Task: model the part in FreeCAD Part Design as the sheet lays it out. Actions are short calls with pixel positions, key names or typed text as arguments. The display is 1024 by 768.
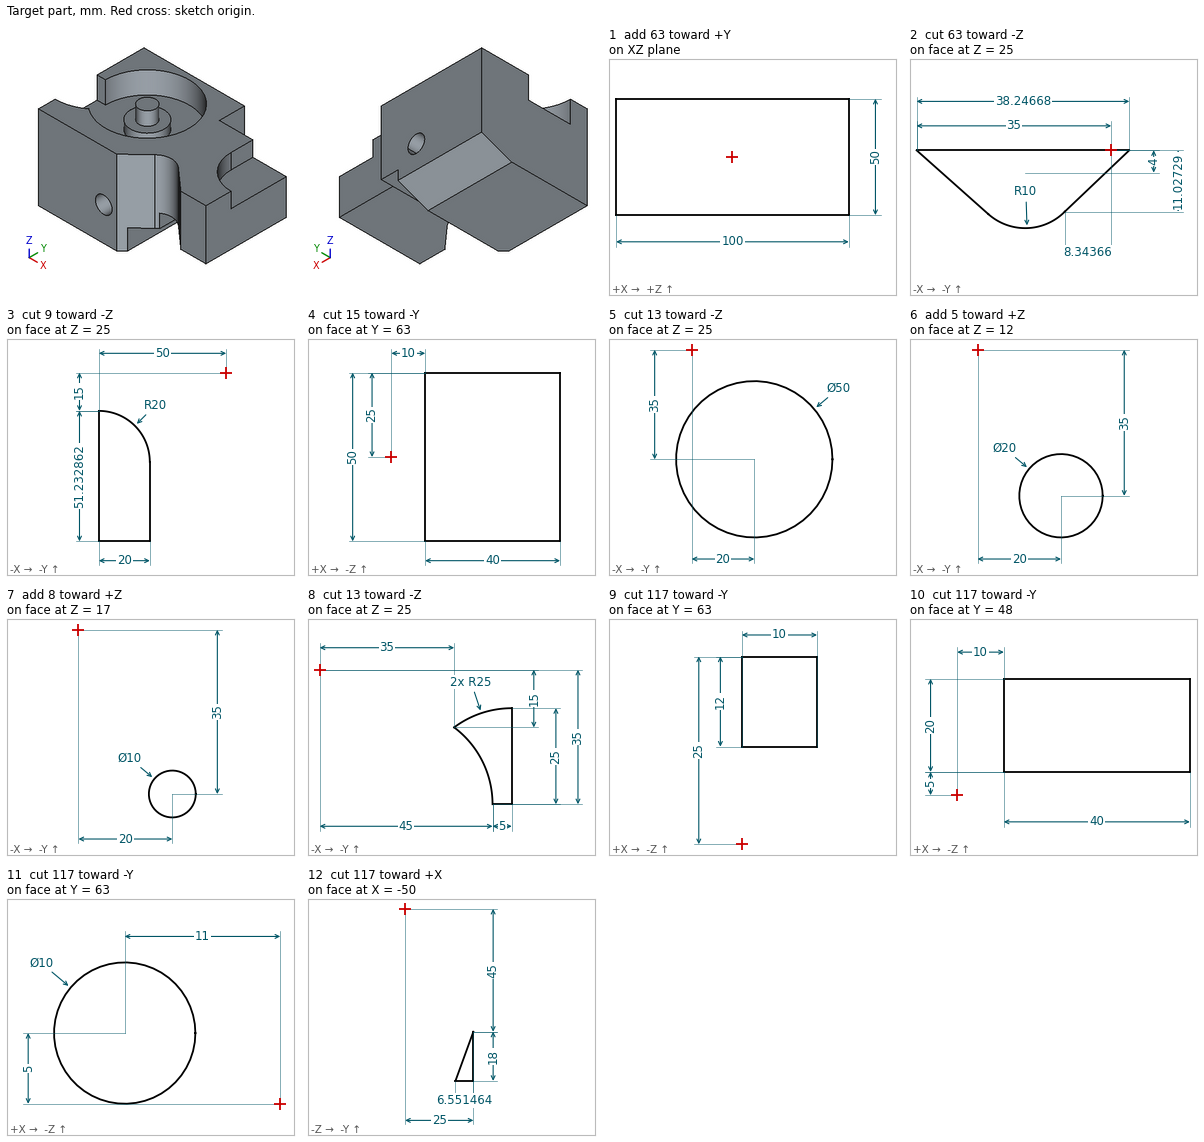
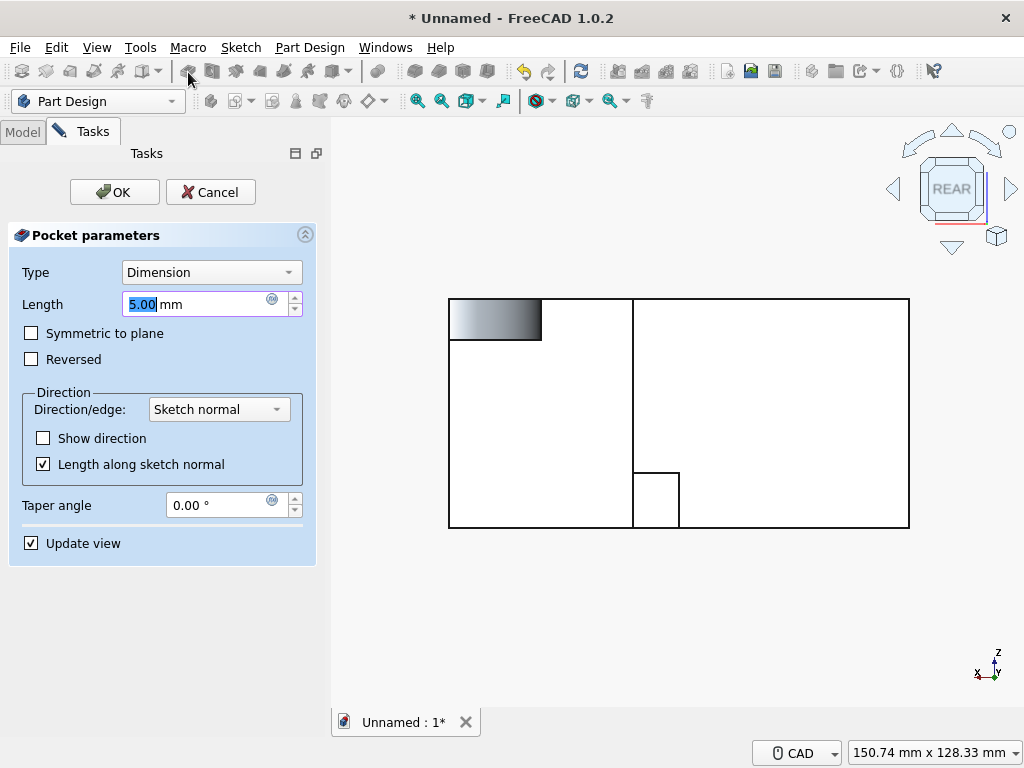
text(117)
key(Tab)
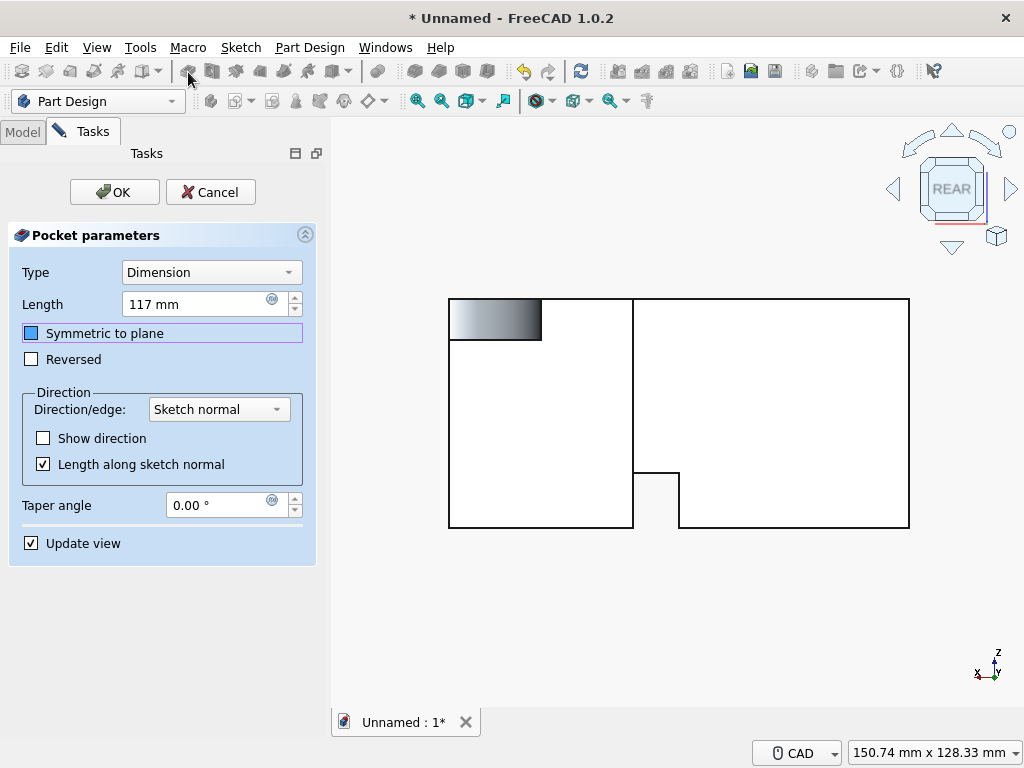
click(115, 192)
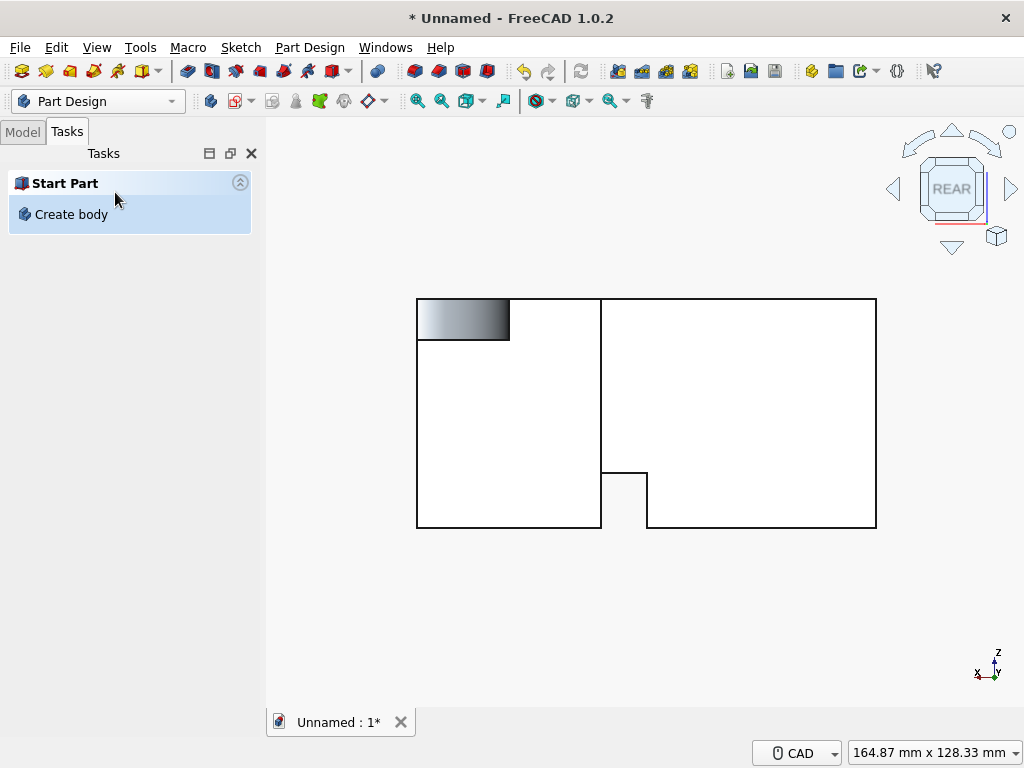
click(509, 445)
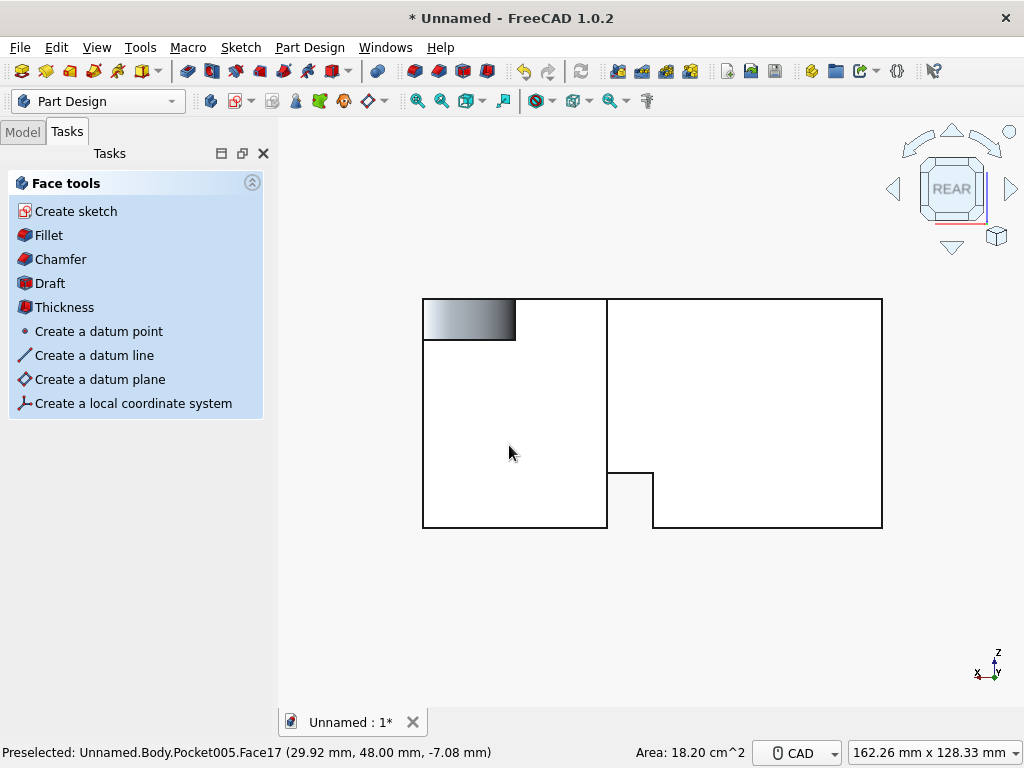
click(236, 102)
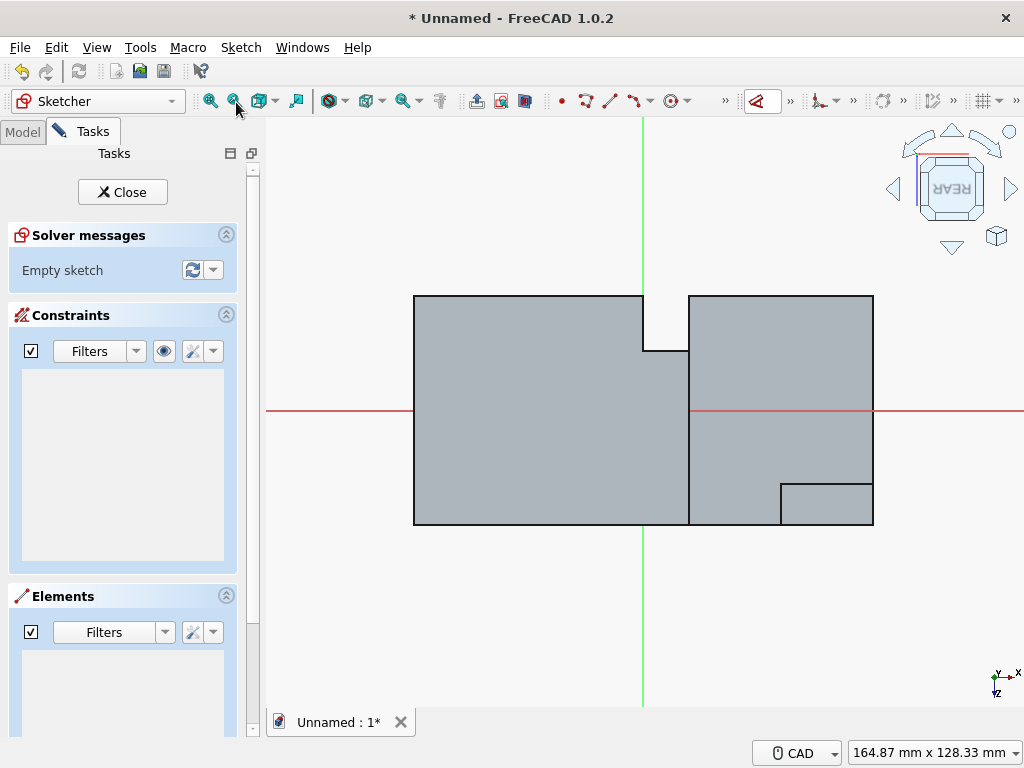
click(526, 102)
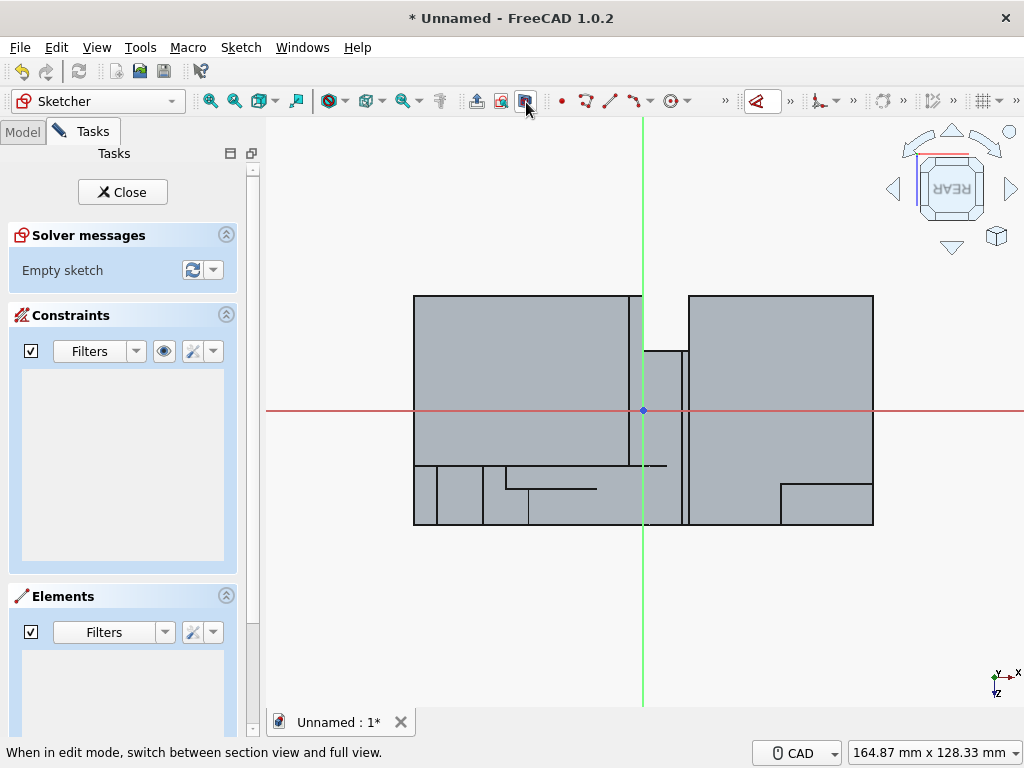
scroll(576, 412, down, 5)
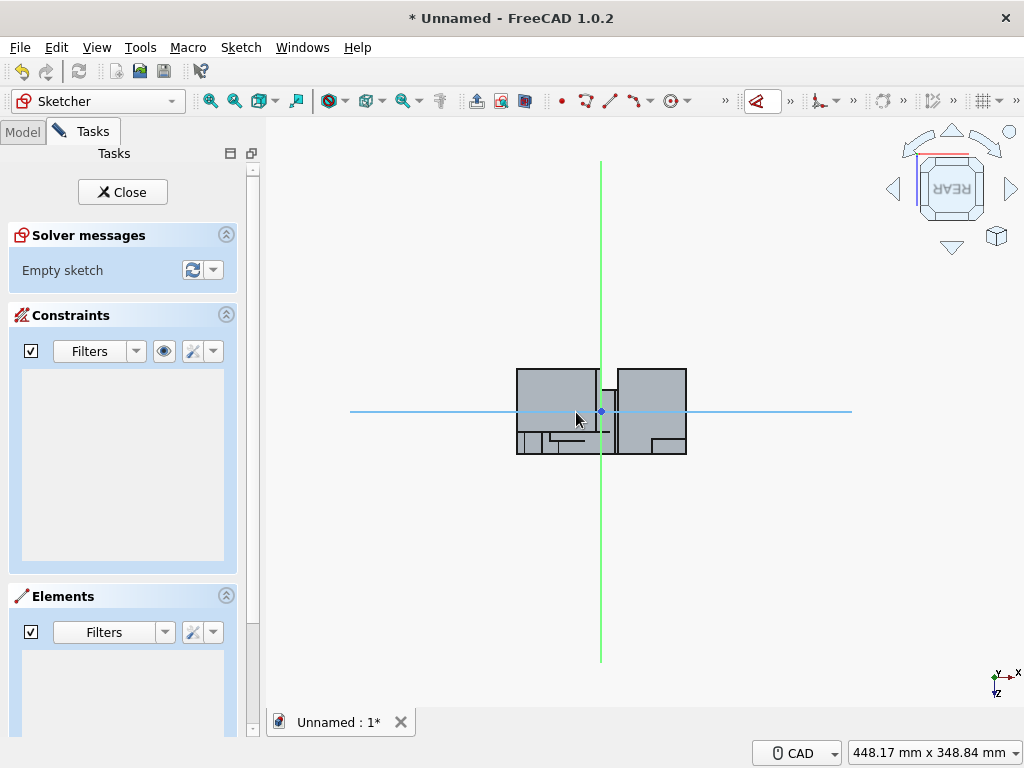
scroll(660, 385, up, 8)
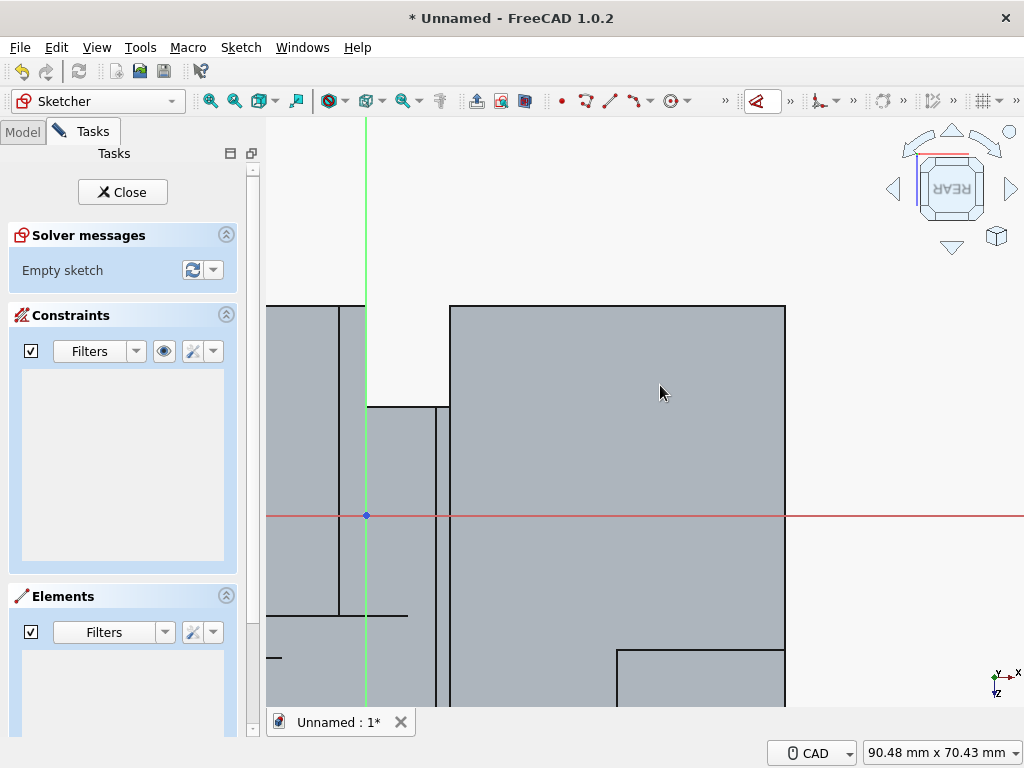
key(g)
key(r)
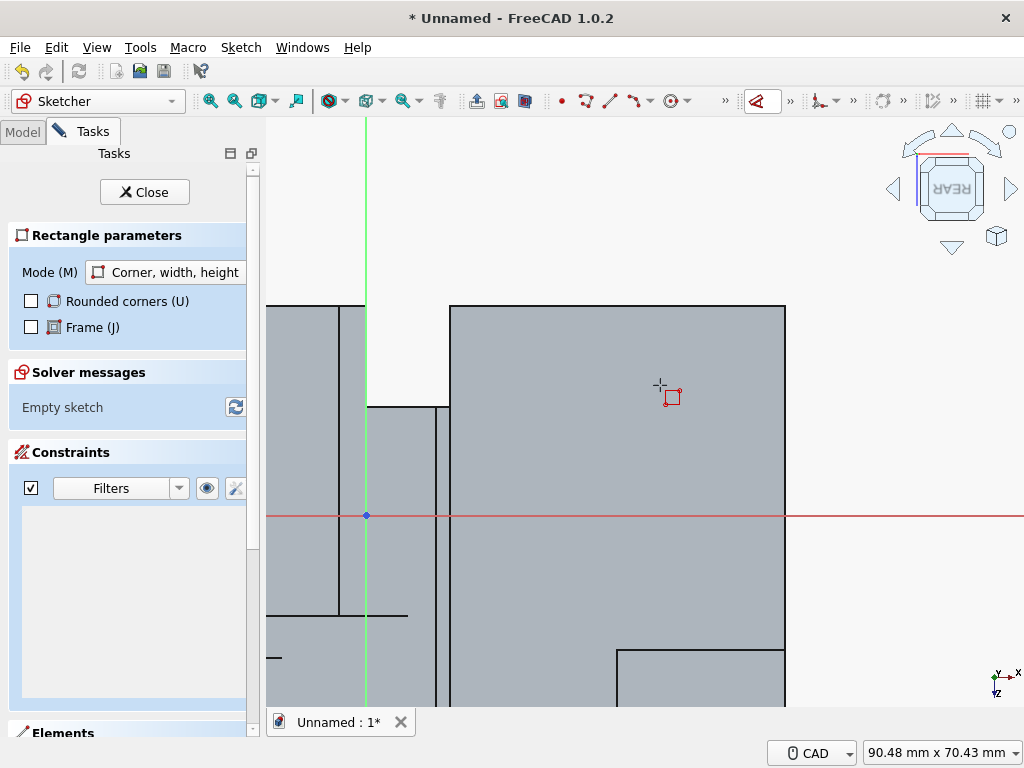
click(450, 306)
click(785, 474)
key(Escape)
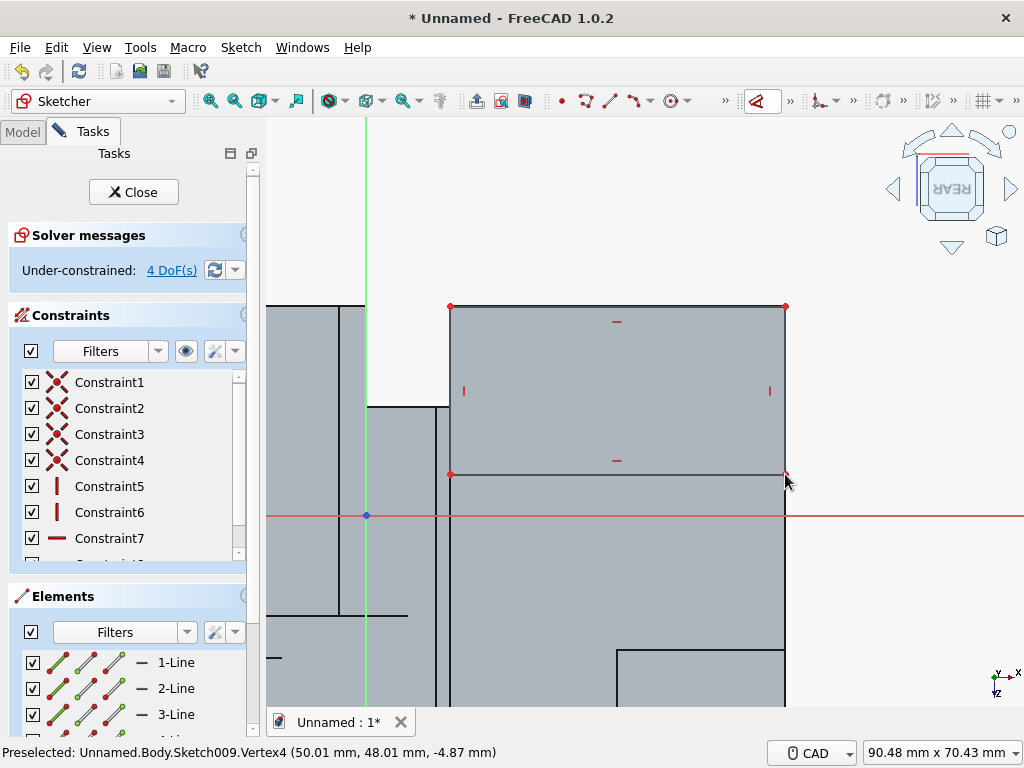
click(450, 357)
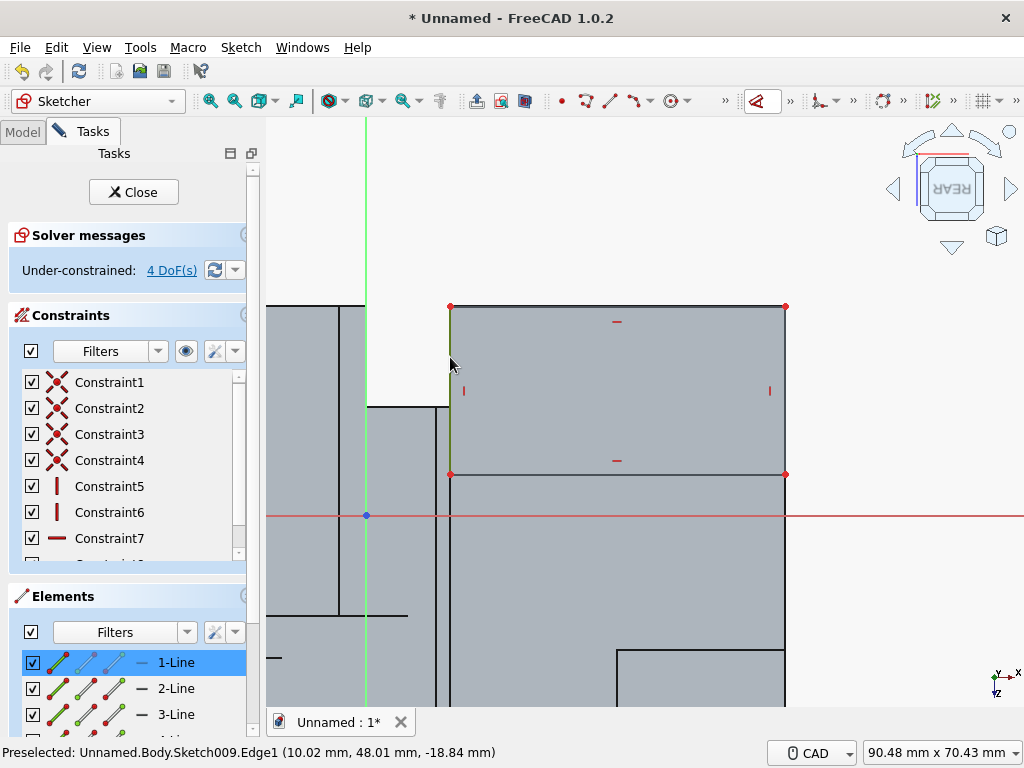
click(776, 102)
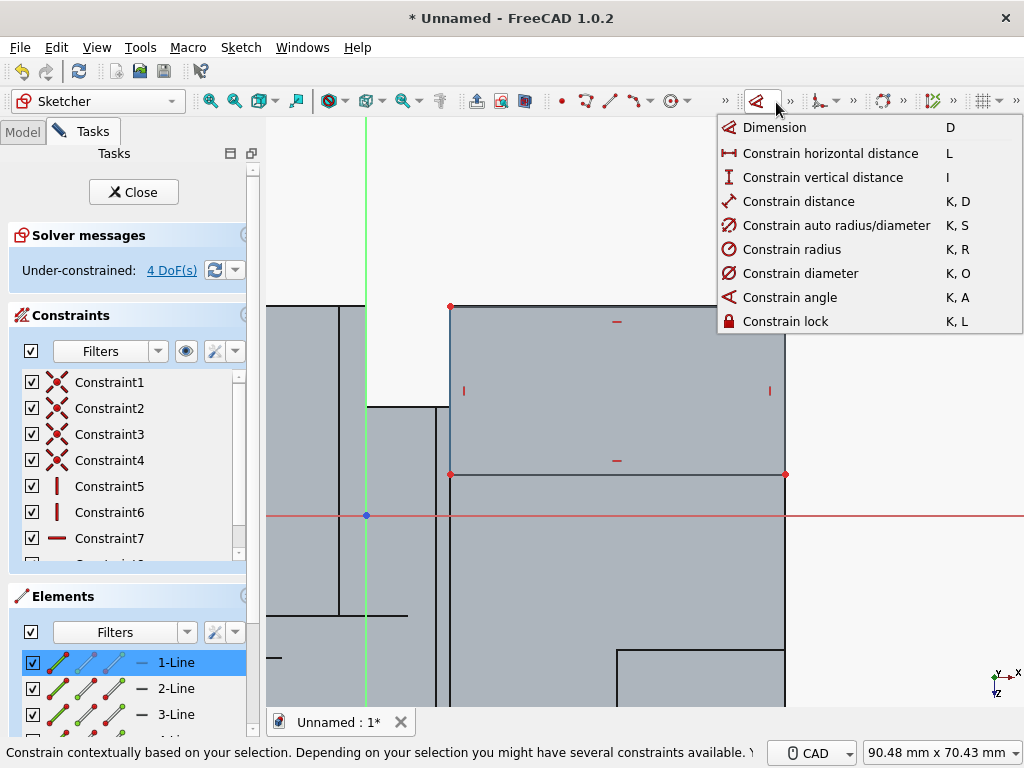
click(870, 177)